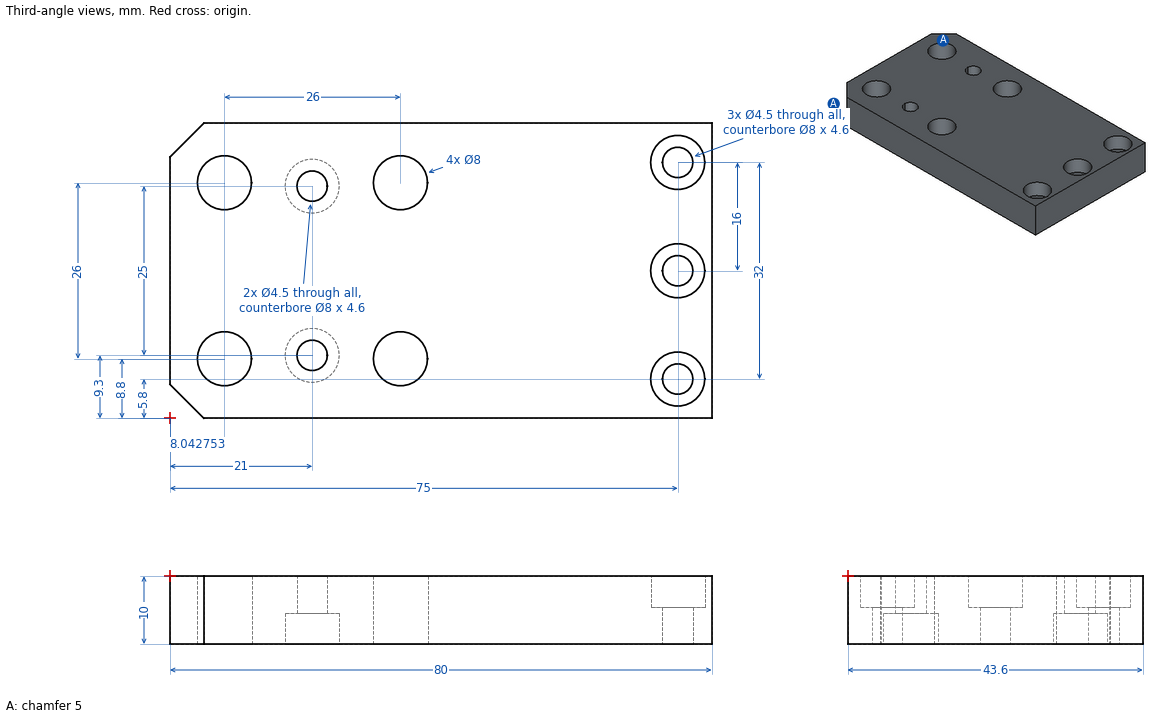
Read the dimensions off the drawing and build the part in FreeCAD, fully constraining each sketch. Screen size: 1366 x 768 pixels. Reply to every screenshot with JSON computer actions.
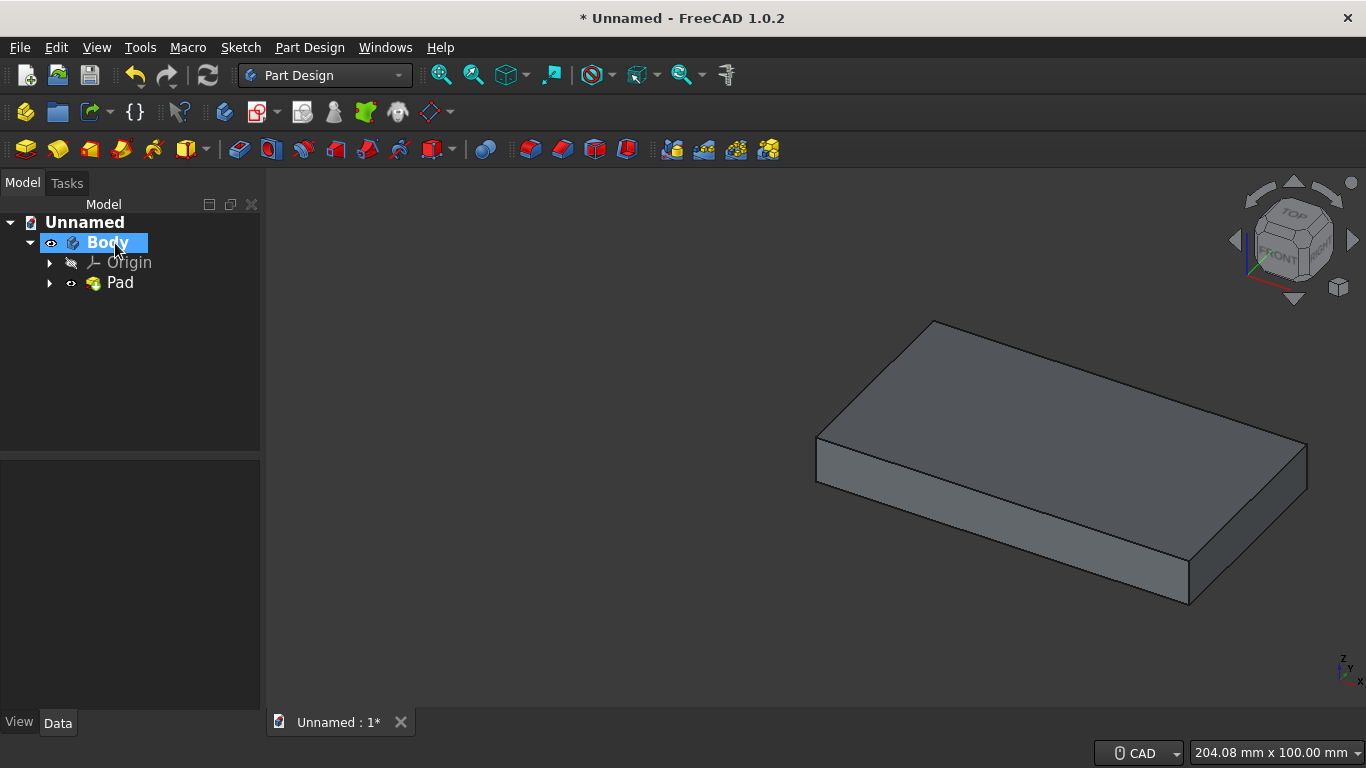
{"action": "key", "text": "0"}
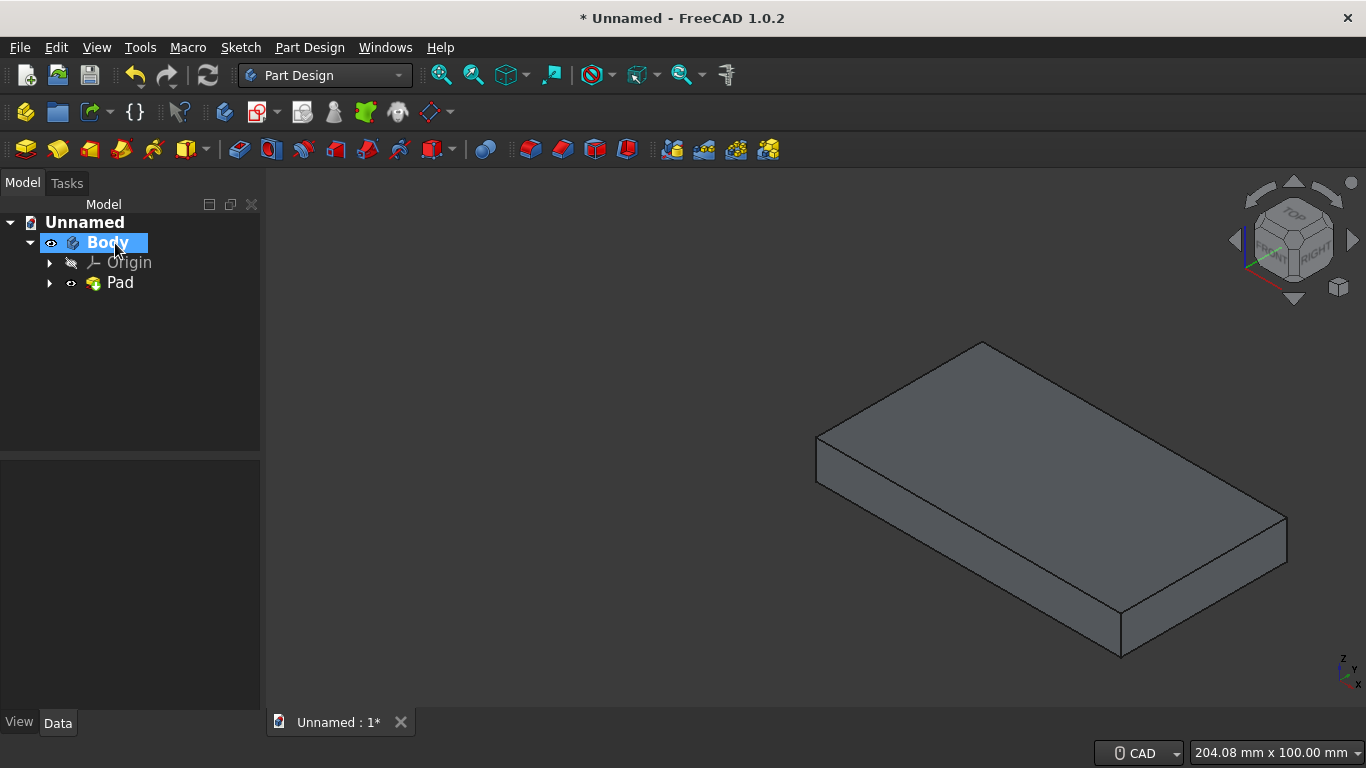
{"action": "key", "text": "2"}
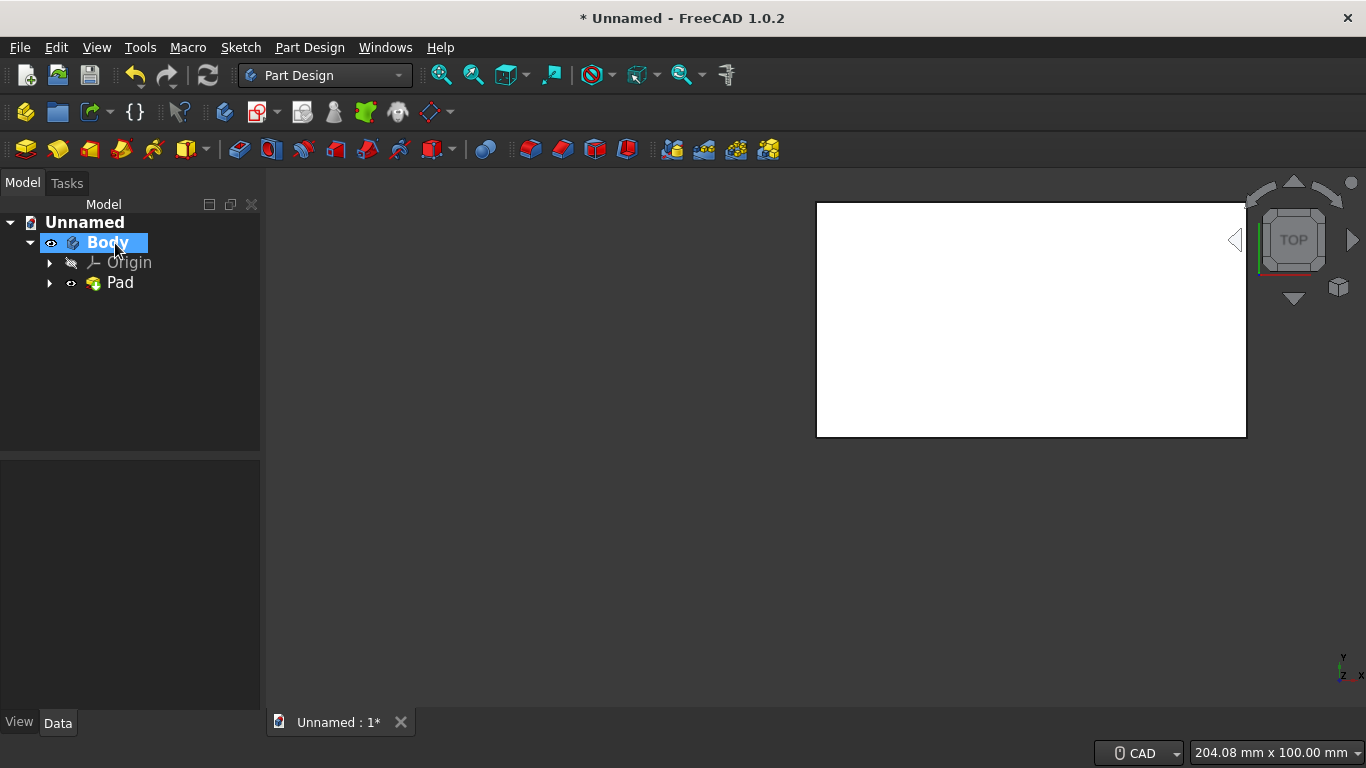
{"action": "left_click", "coordinate": [442, 76]}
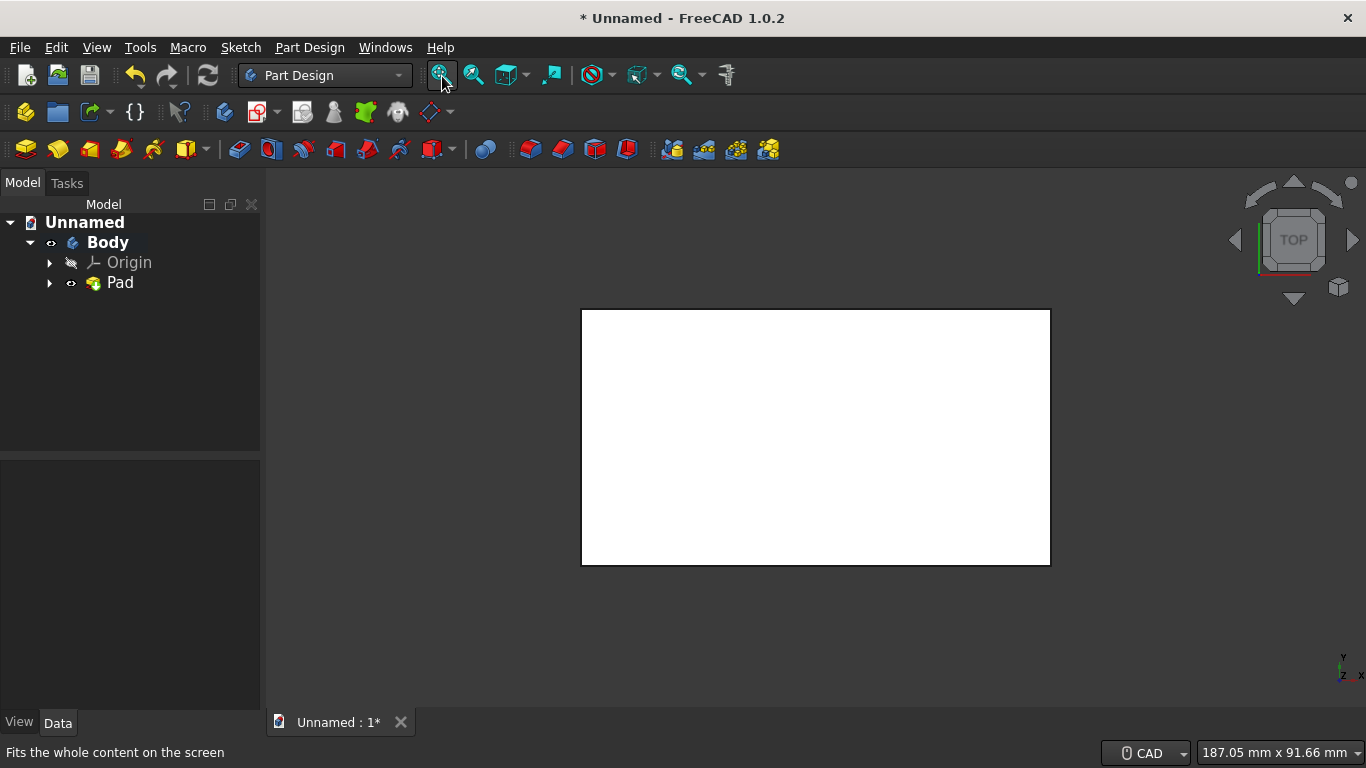
{"action": "key", "text": "1"}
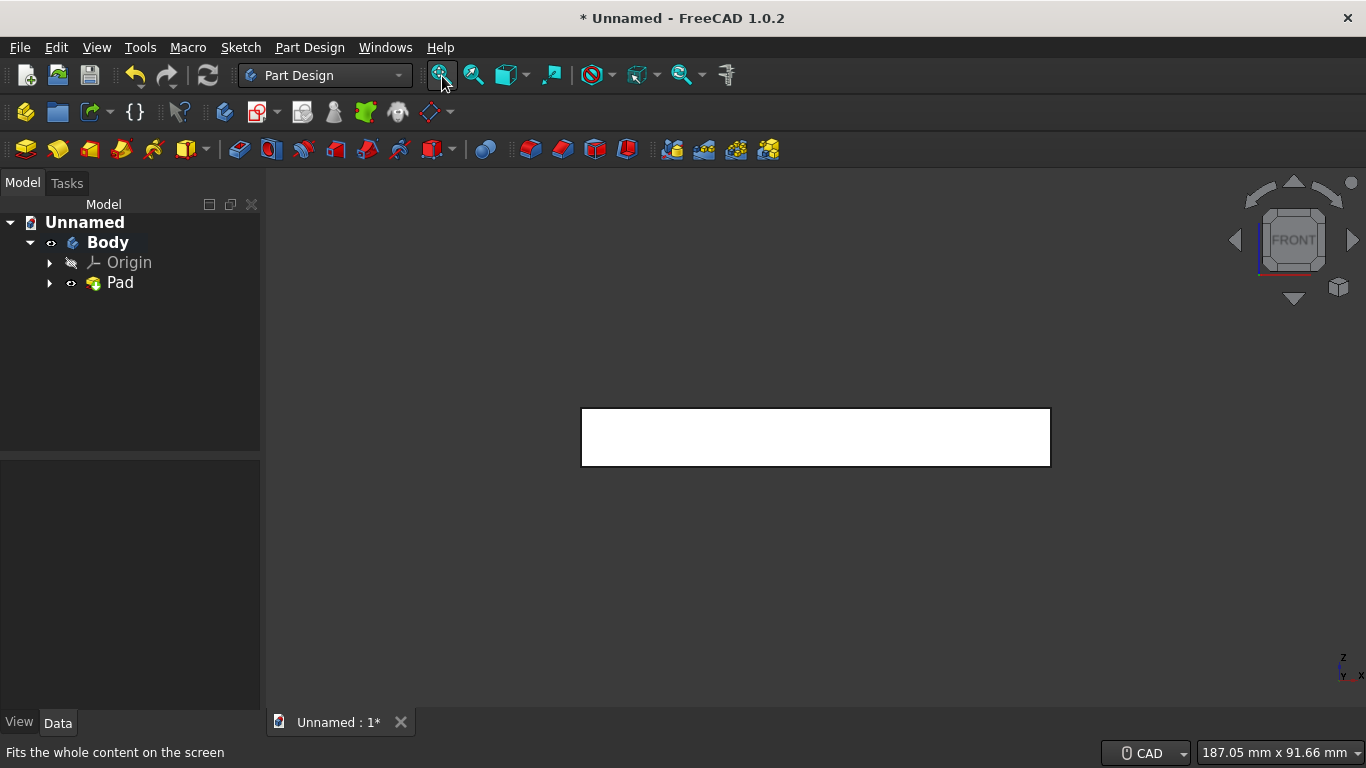
{"action": "left_click", "coordinate": [442, 76]}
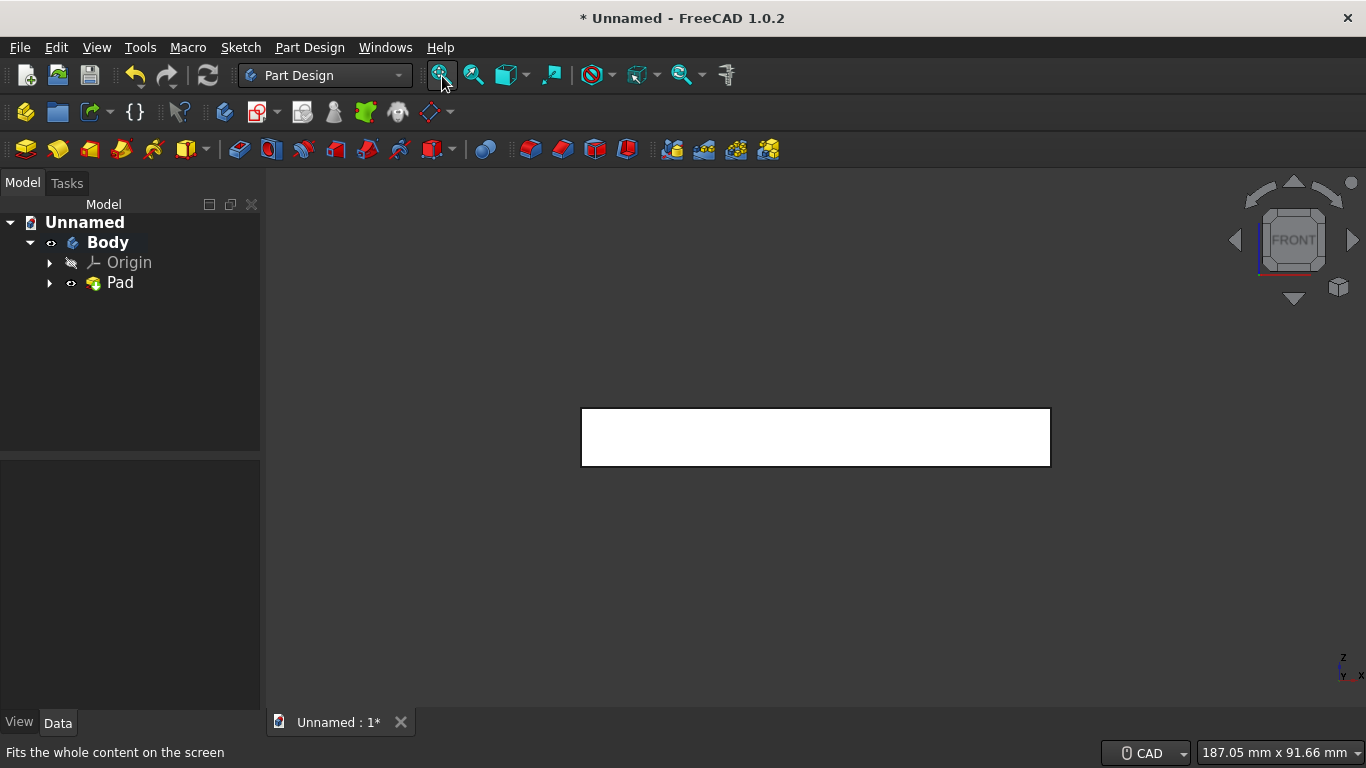
{"action": "left_click", "coordinate": [581, 431]}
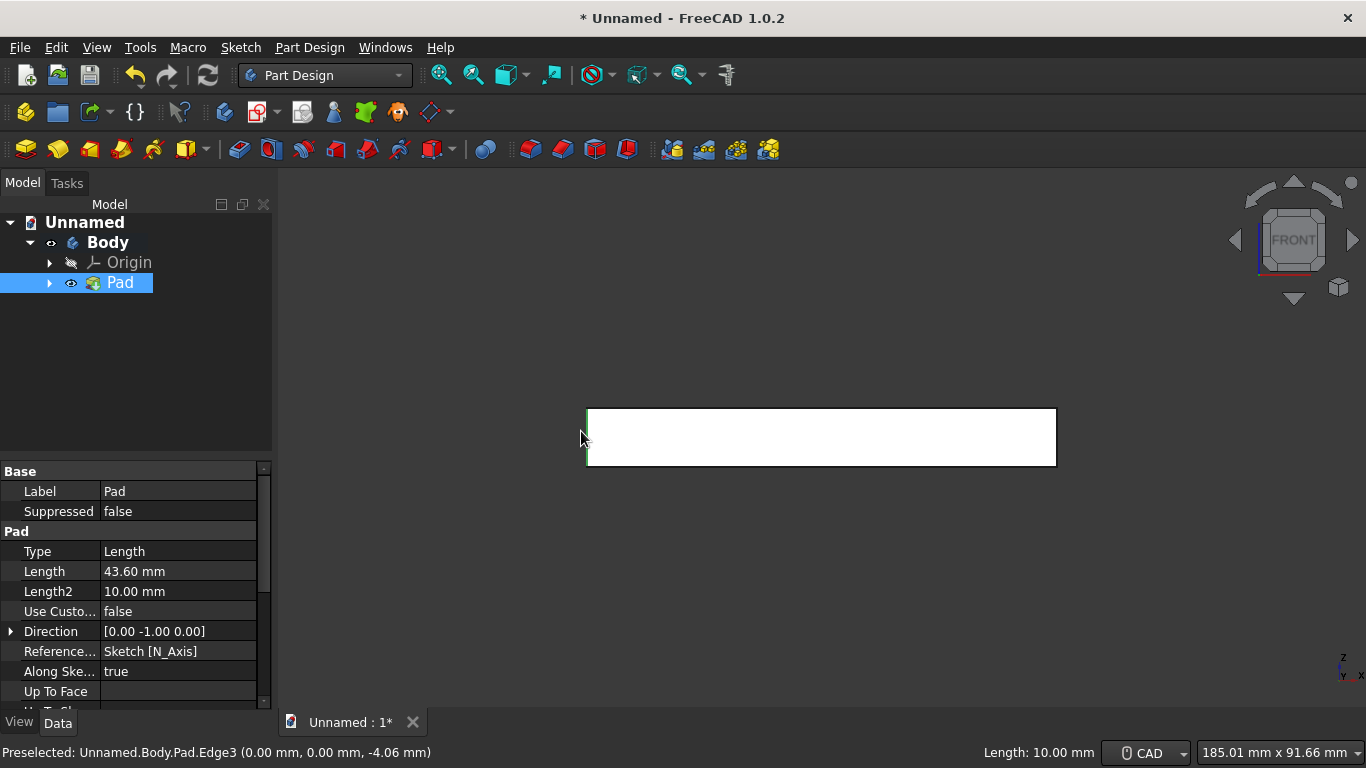
{"action": "key", "text": "3"}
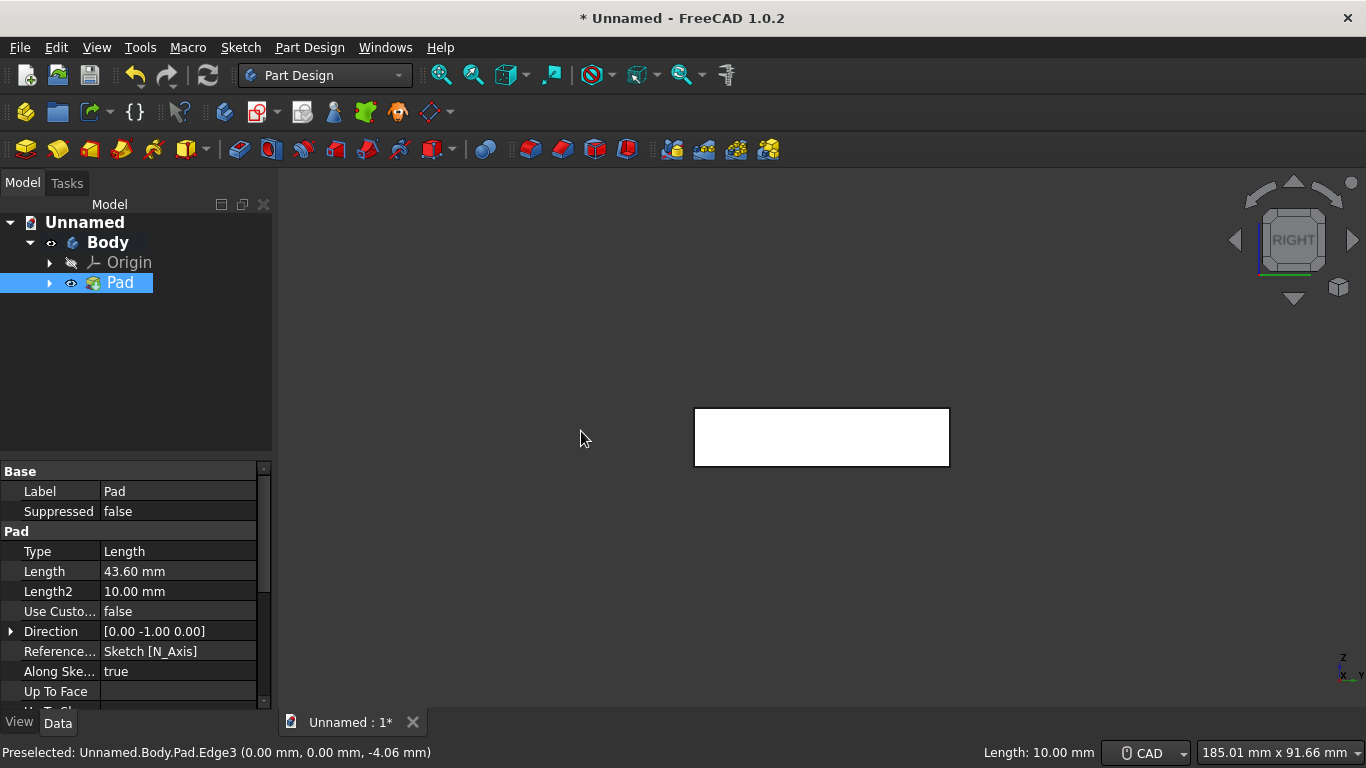
{"action": "left_click", "coordinate": [442, 76]}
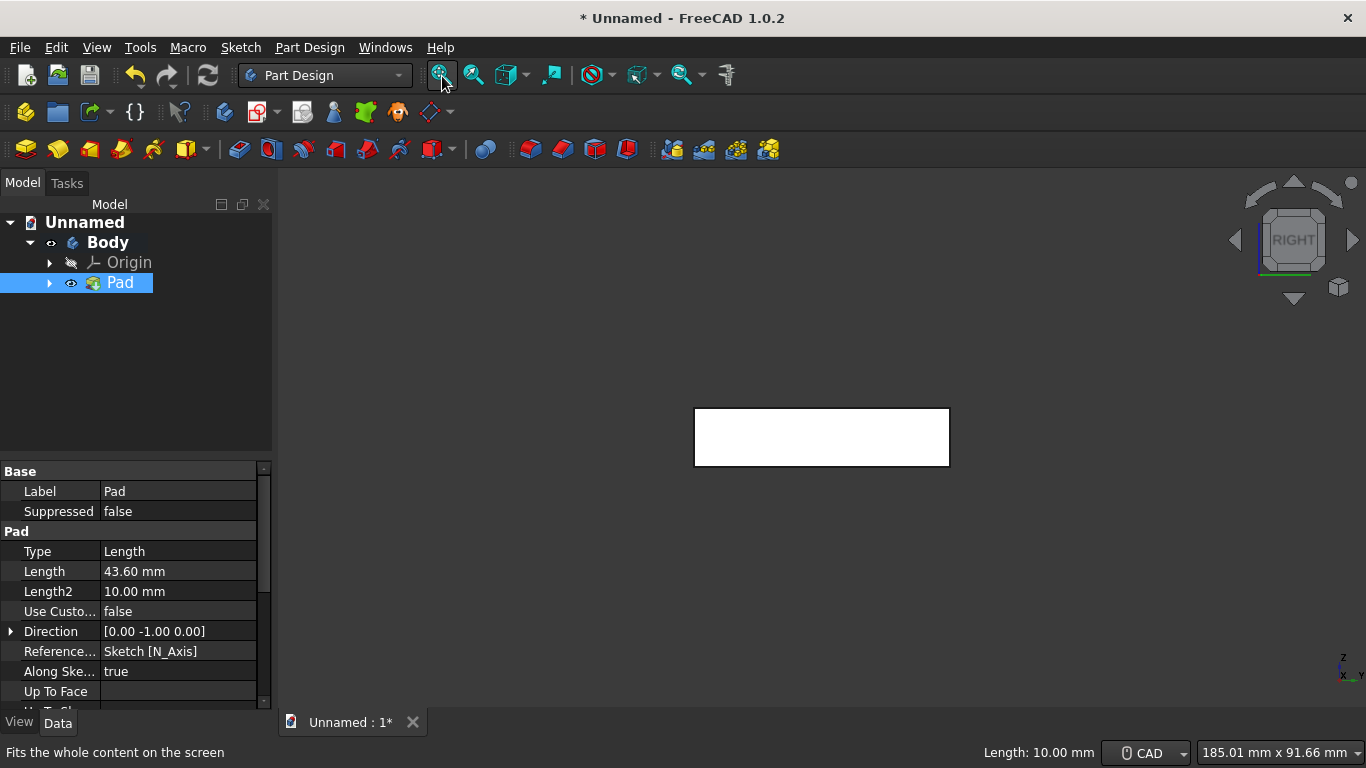
{"action": "key", "text": "5"}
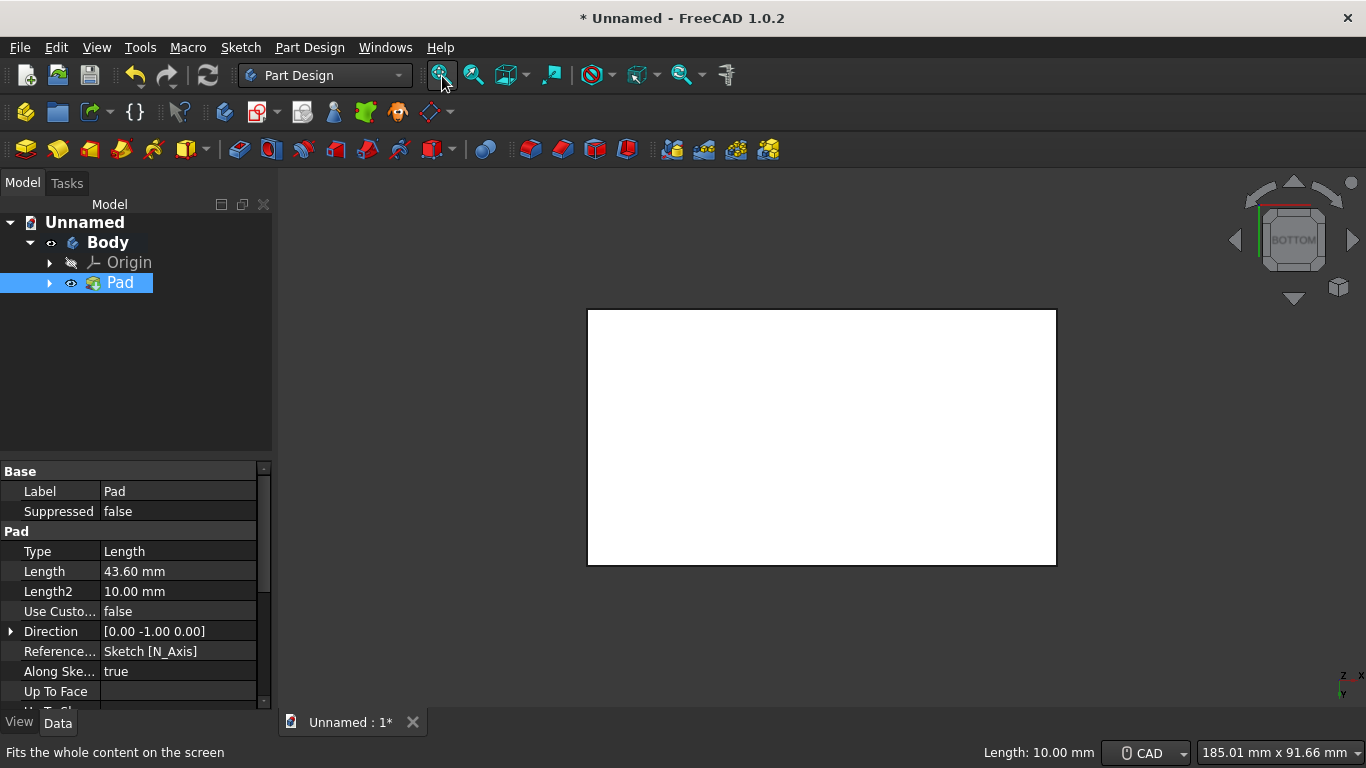
{"action": "key", "text": "4"}